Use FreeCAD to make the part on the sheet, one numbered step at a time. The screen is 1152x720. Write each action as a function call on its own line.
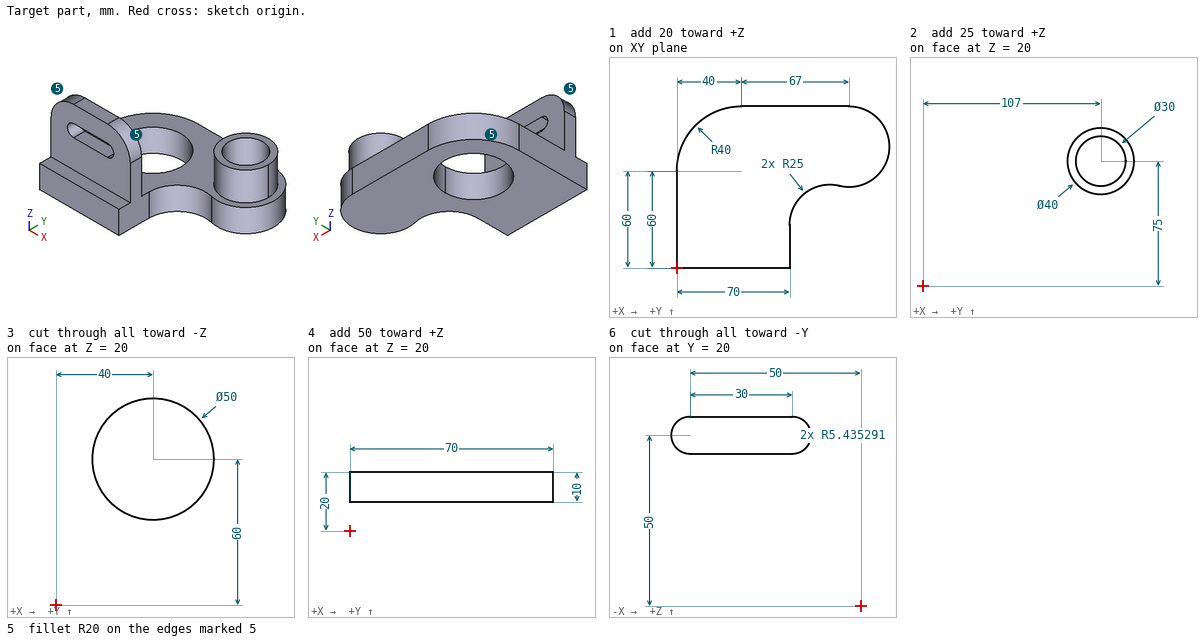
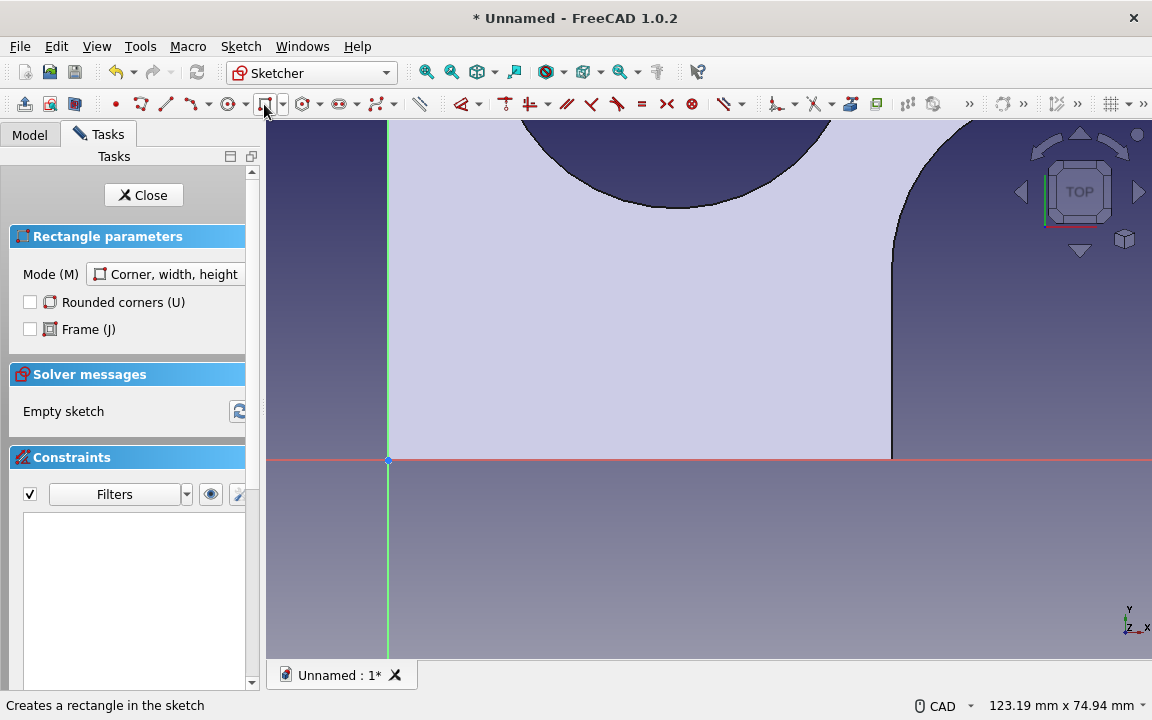
click(388, 316)
move(892, 388)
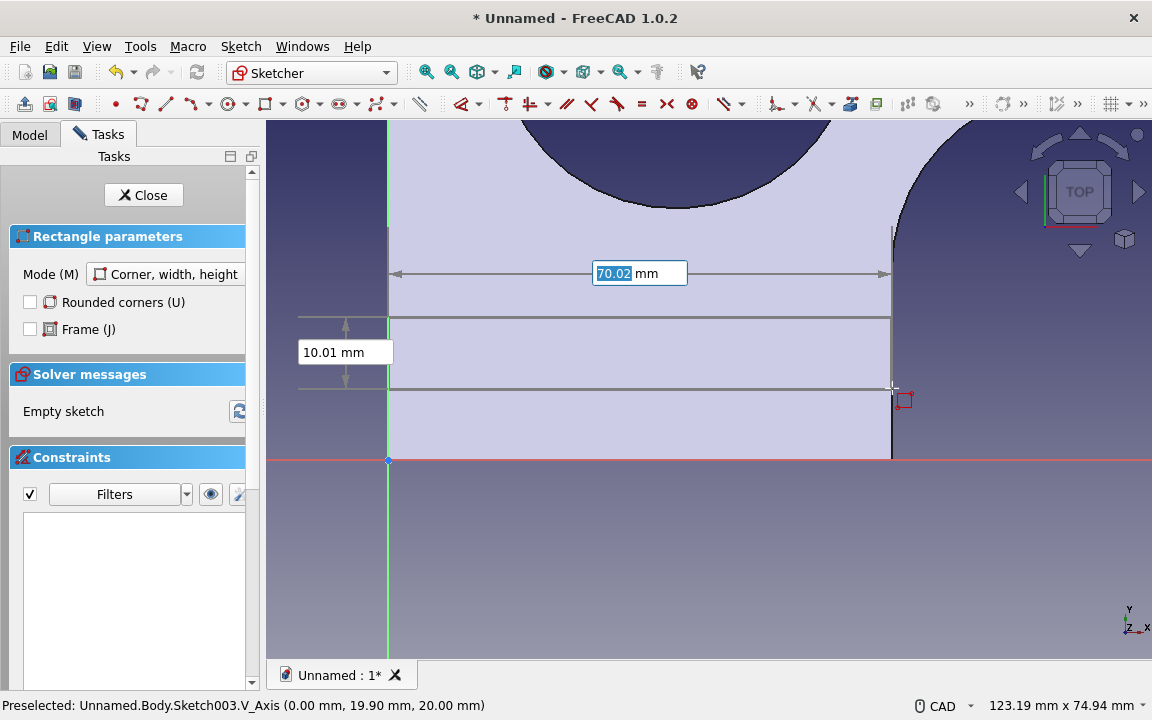
text(70)
key(Tab)
text(10)
key(Return)
key(Escape)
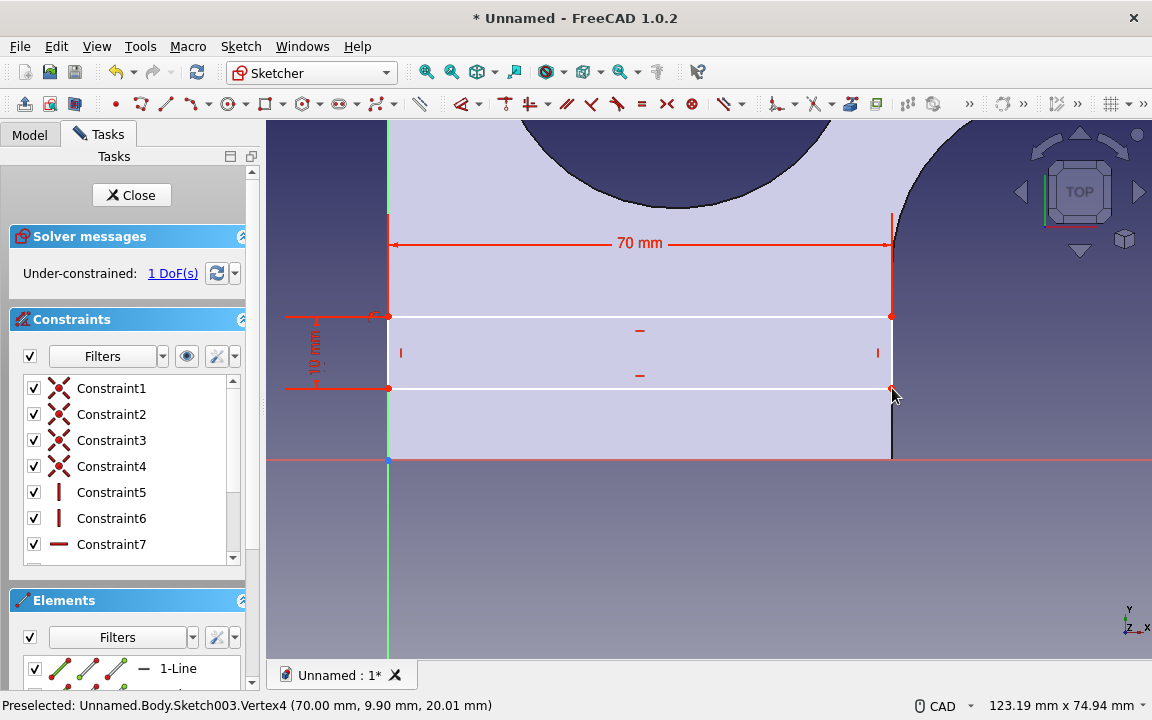
click(460, 104)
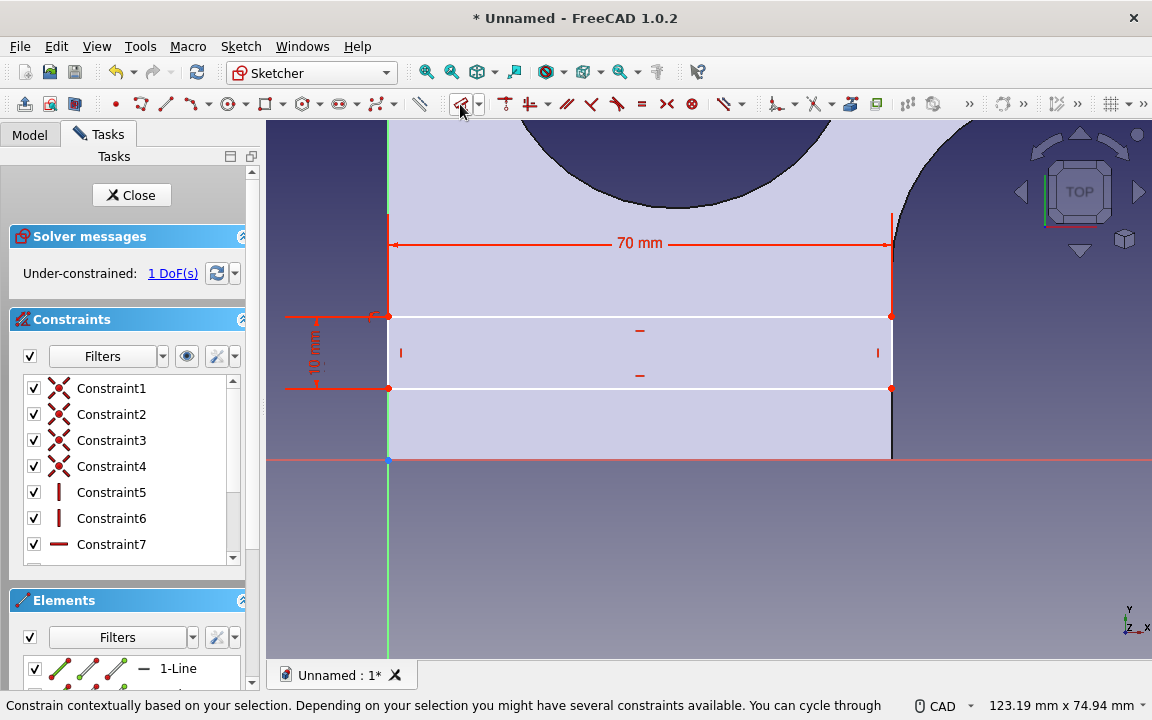
click(388, 317)
click(354, 389)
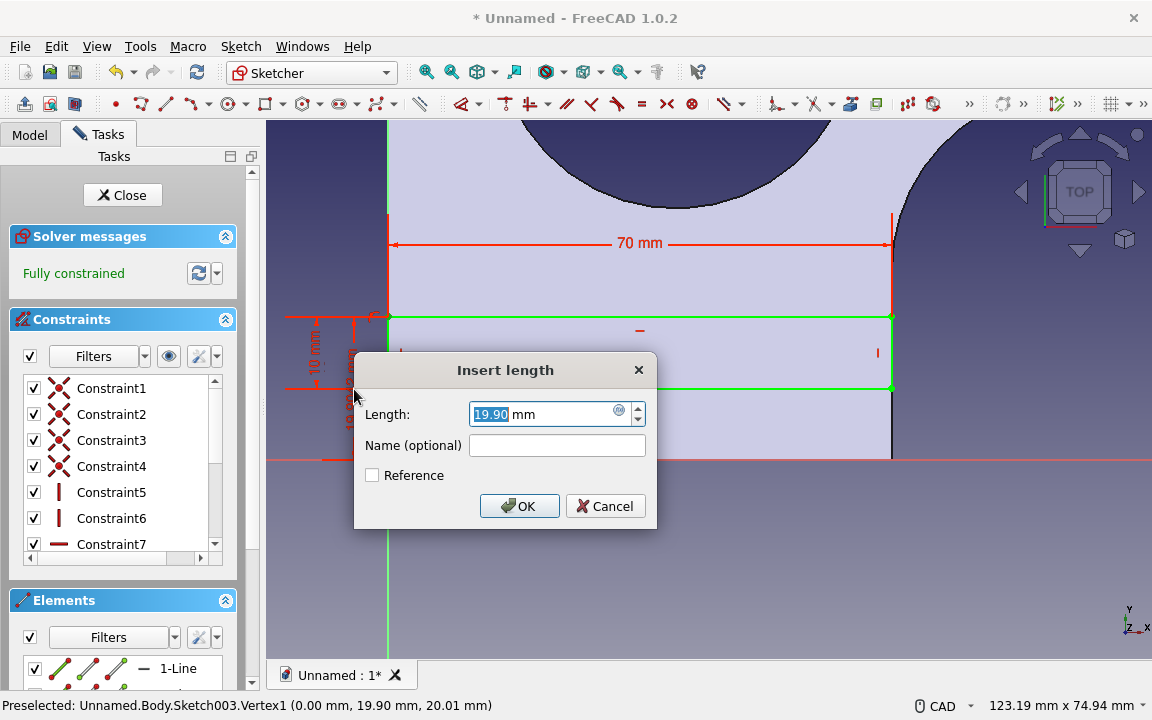
text(20)
key(Return)
key(Escape)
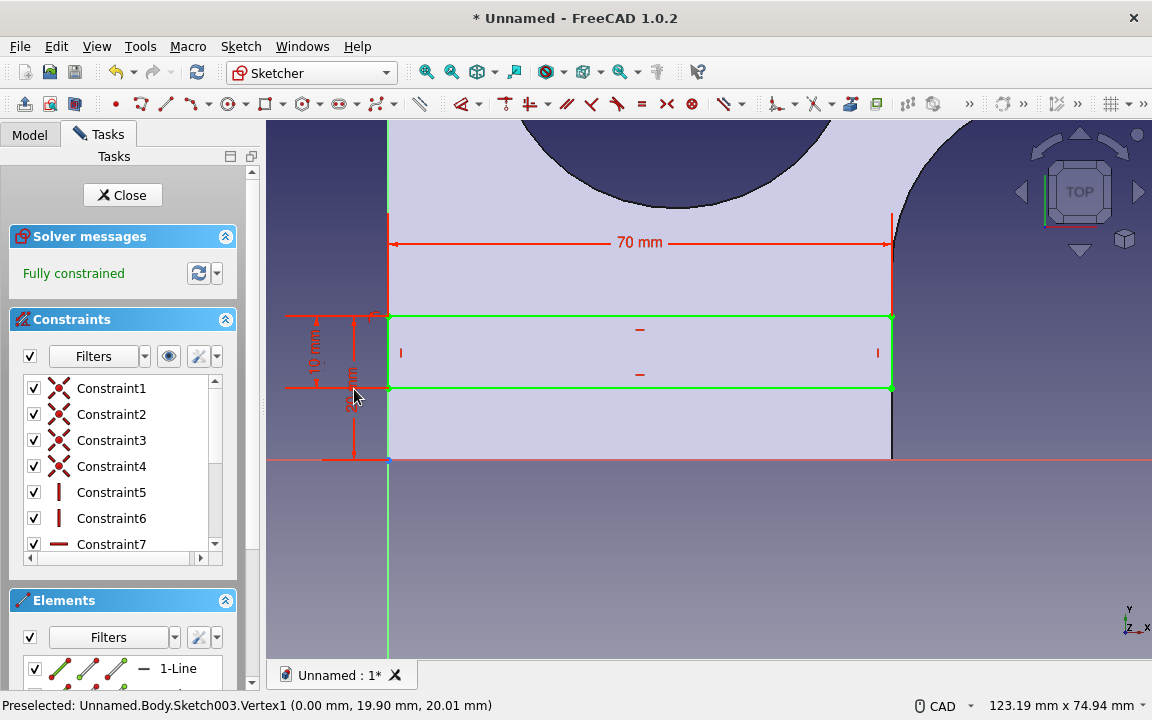
click(123, 195)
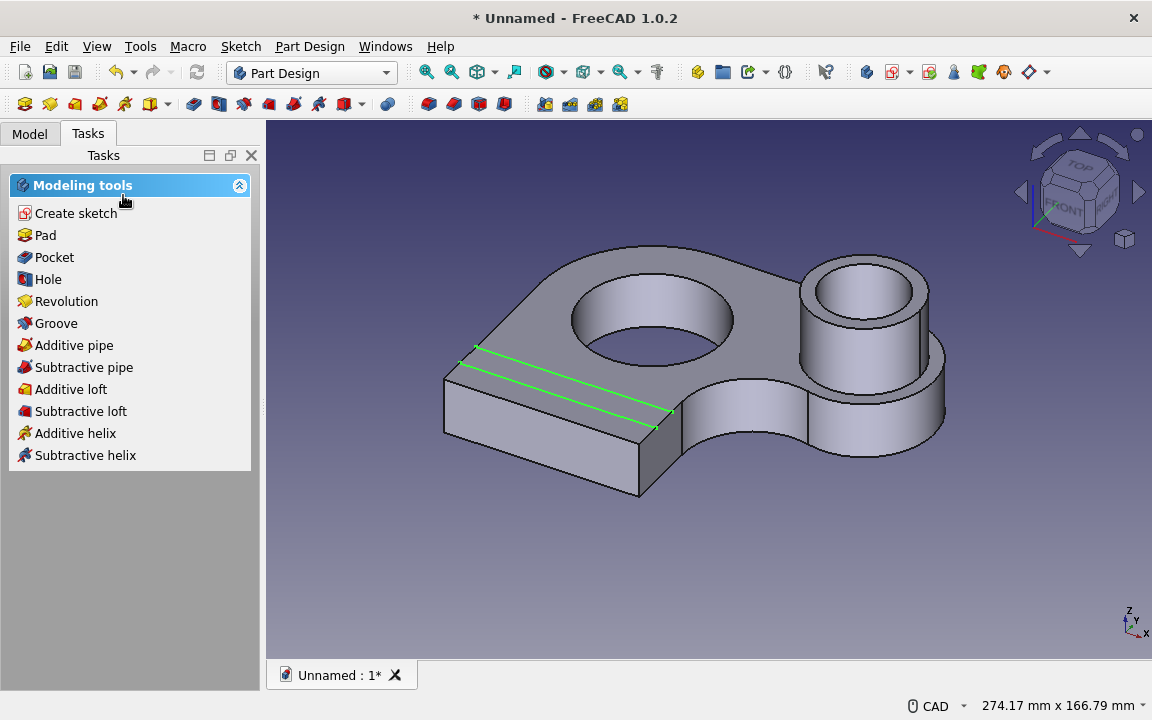
click(25, 104)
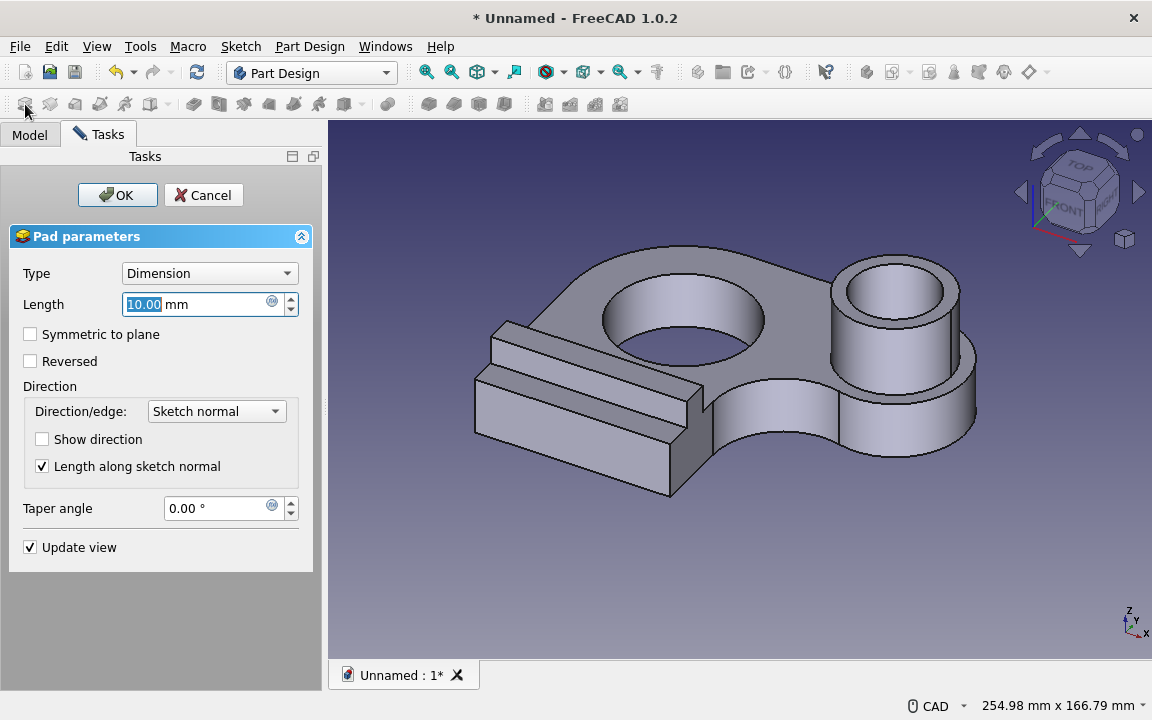
text(50)
key(Tab)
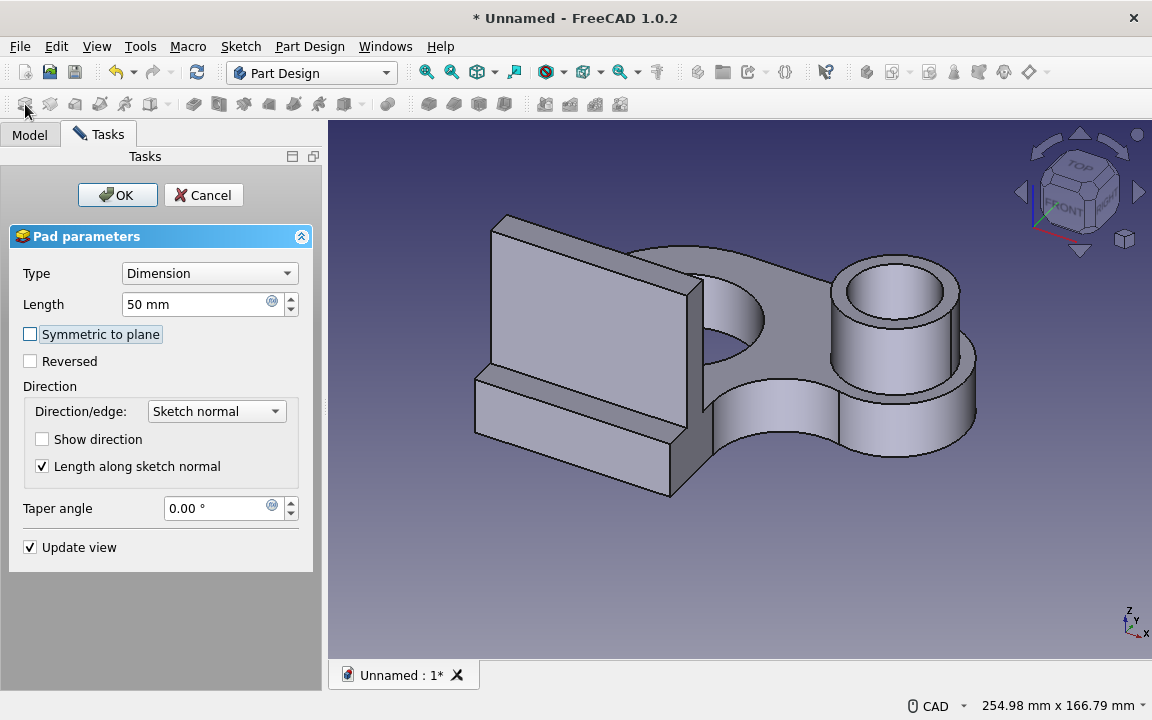
click(118, 195)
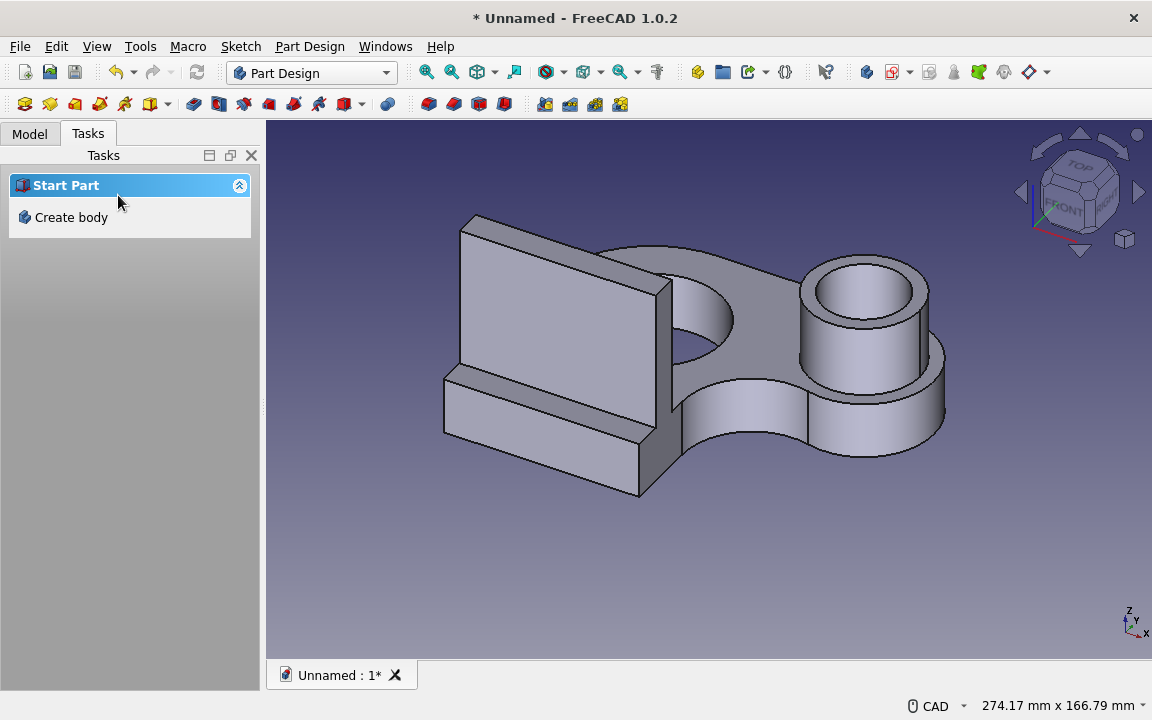
click(427, 72)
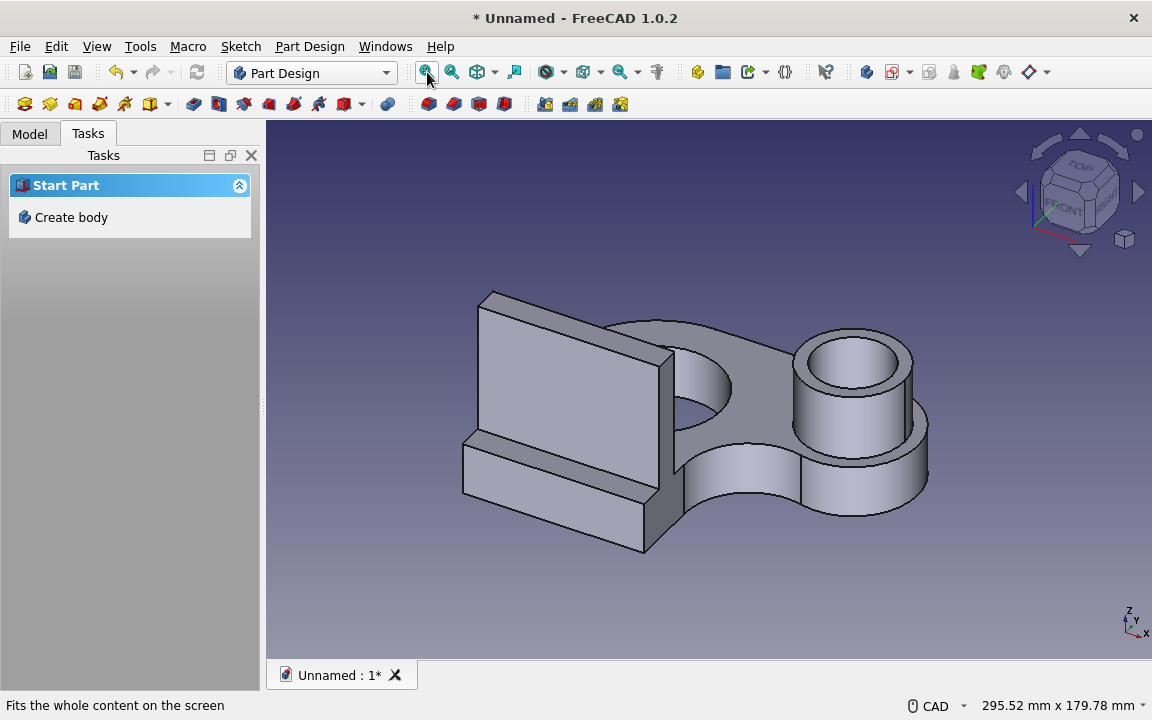
click(667, 358)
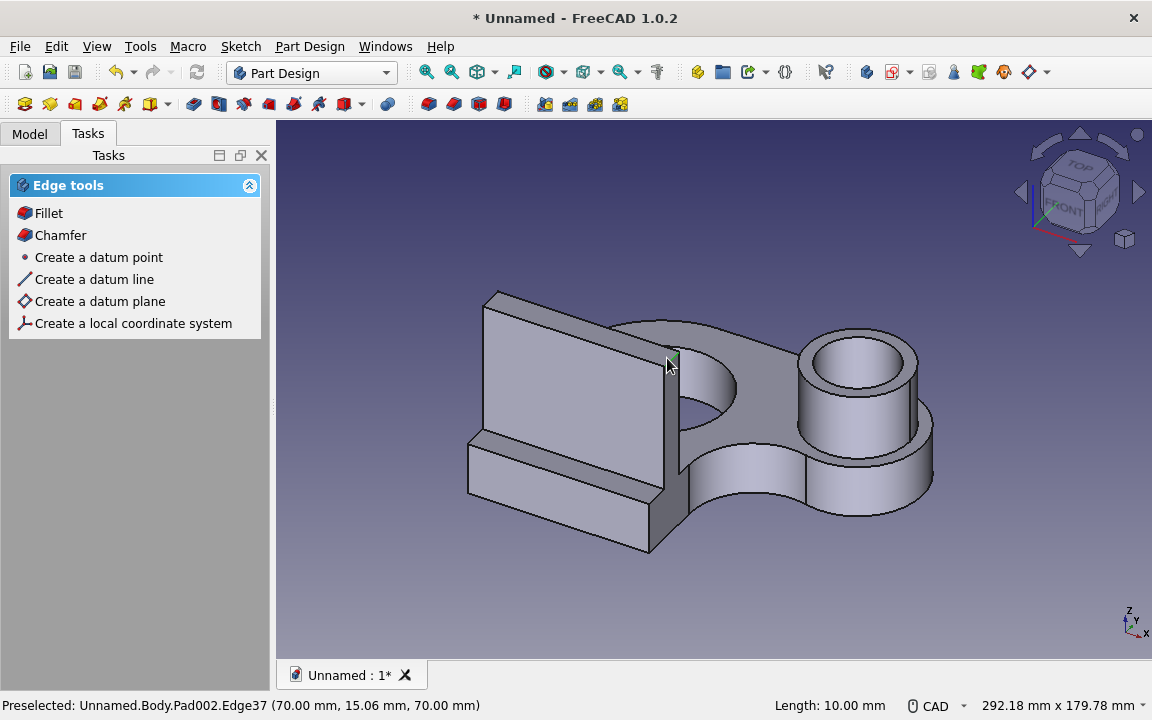
key(0)